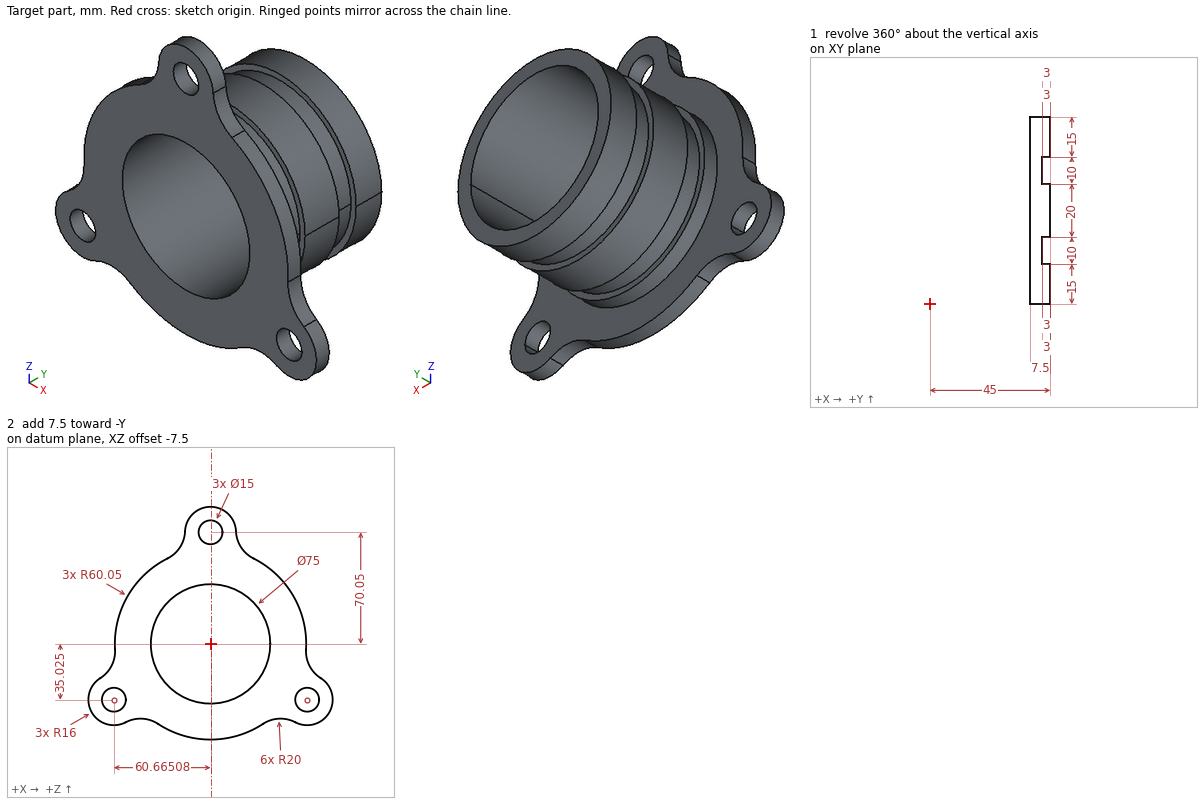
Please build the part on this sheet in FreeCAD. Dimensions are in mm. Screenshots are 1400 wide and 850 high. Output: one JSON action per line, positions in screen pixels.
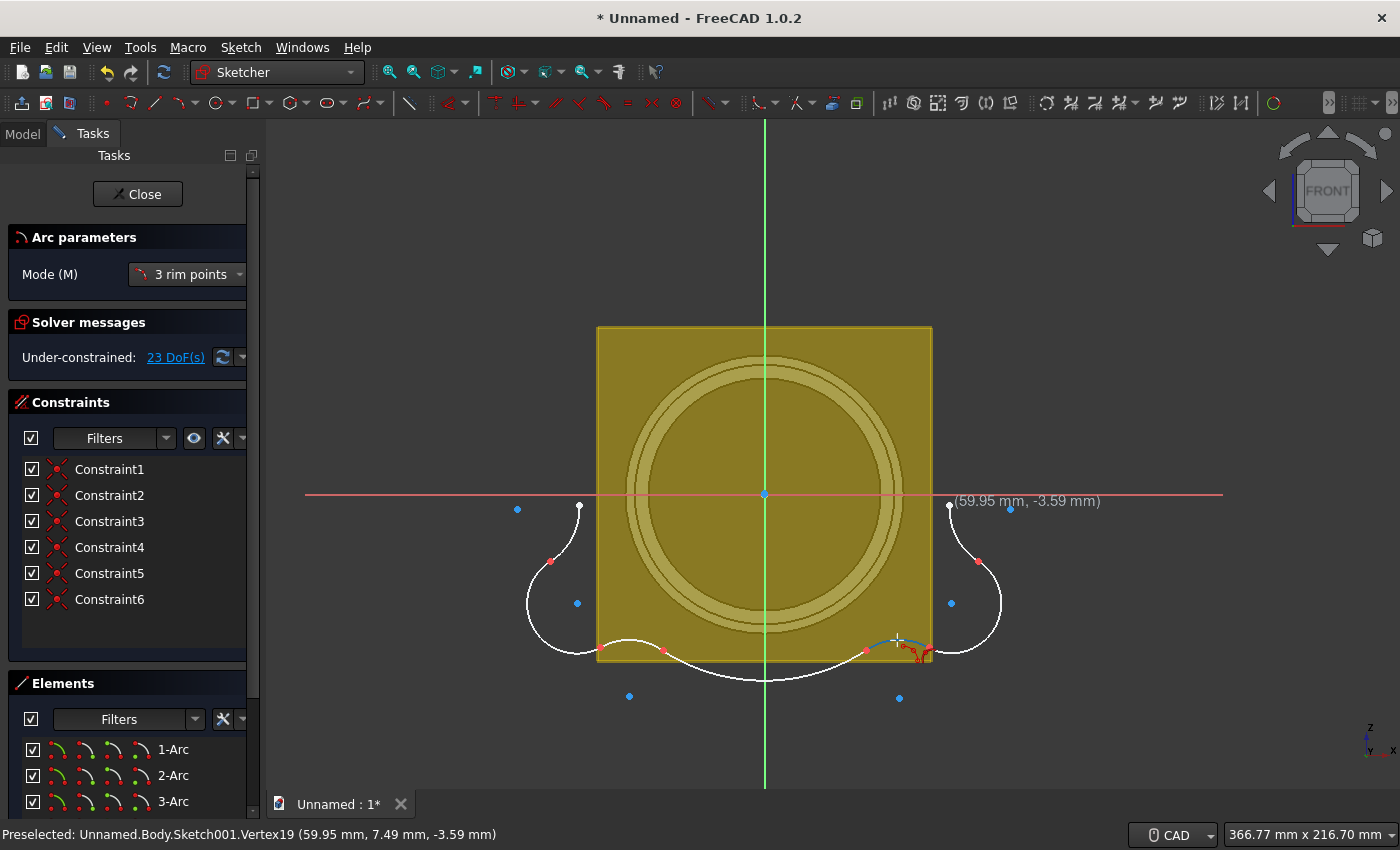
{"action": "left_click", "coordinate": [848, 329]}
{"action": "left_click", "coordinate": [925, 402]}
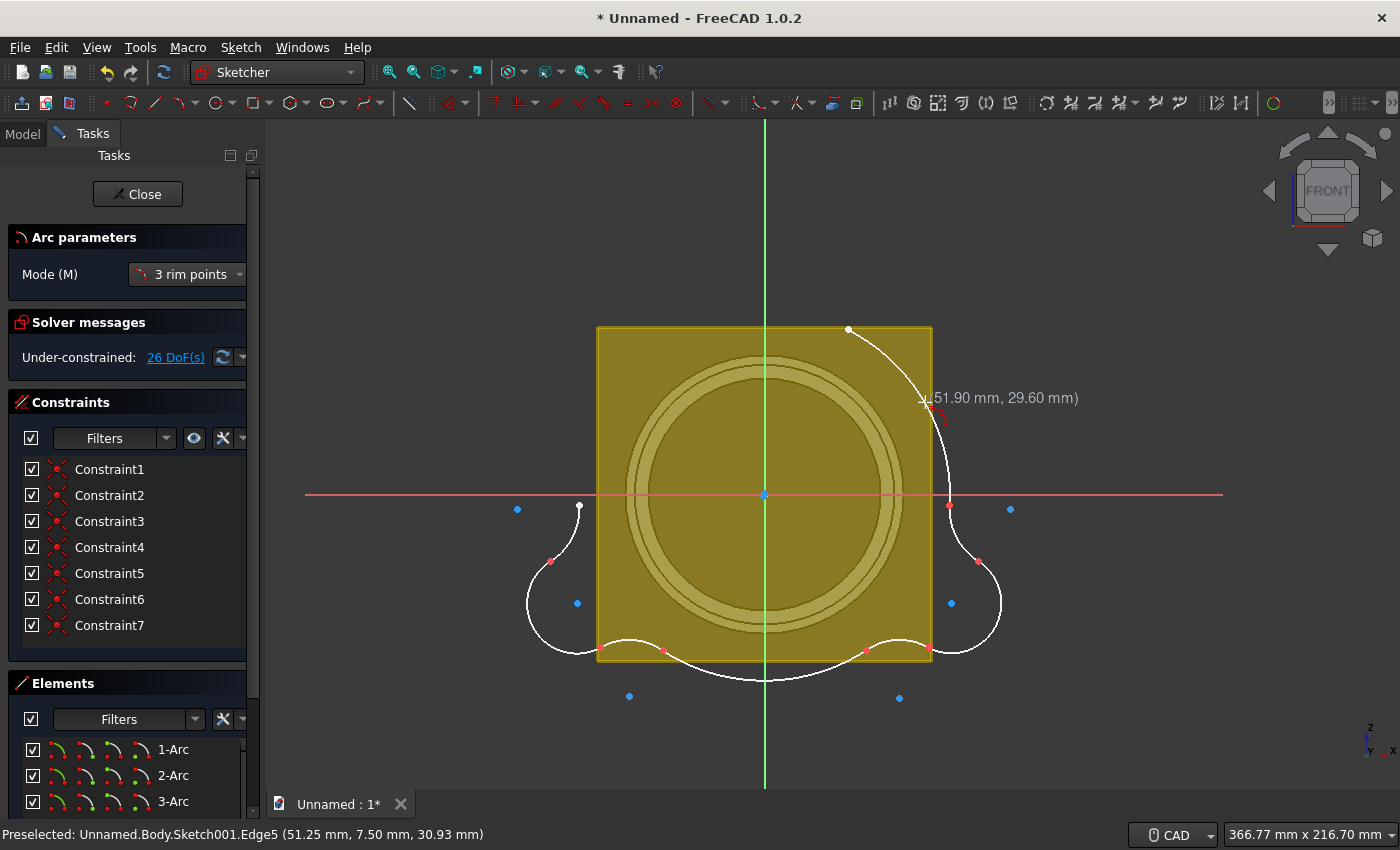
{"action": "left_click", "coordinate": [848, 330]}
{"action": "left_click", "coordinate": [814, 276]}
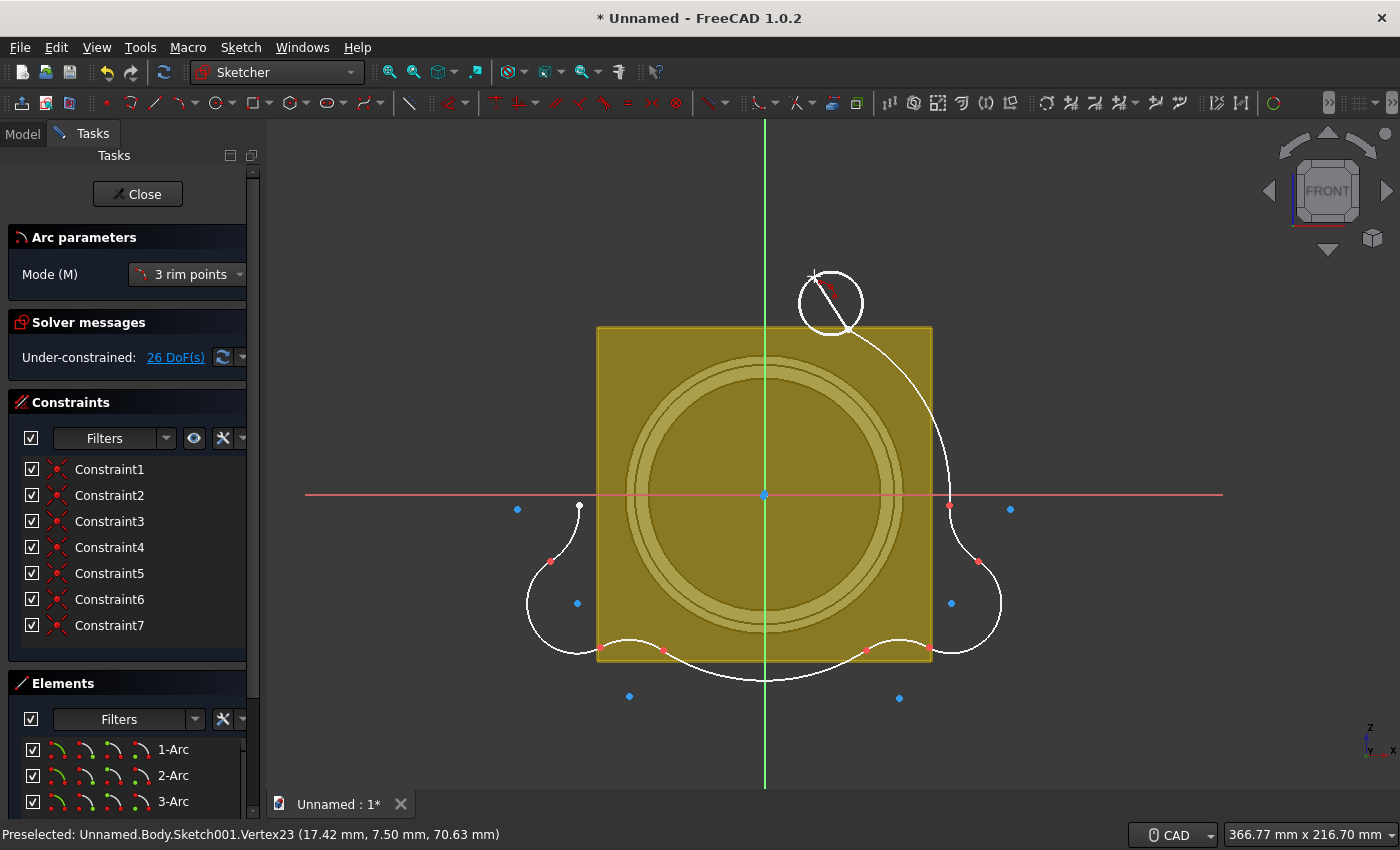
{"action": "scroll", "coordinate": [824, 307], "scroll_direction": "up", "scroll_amount": 4}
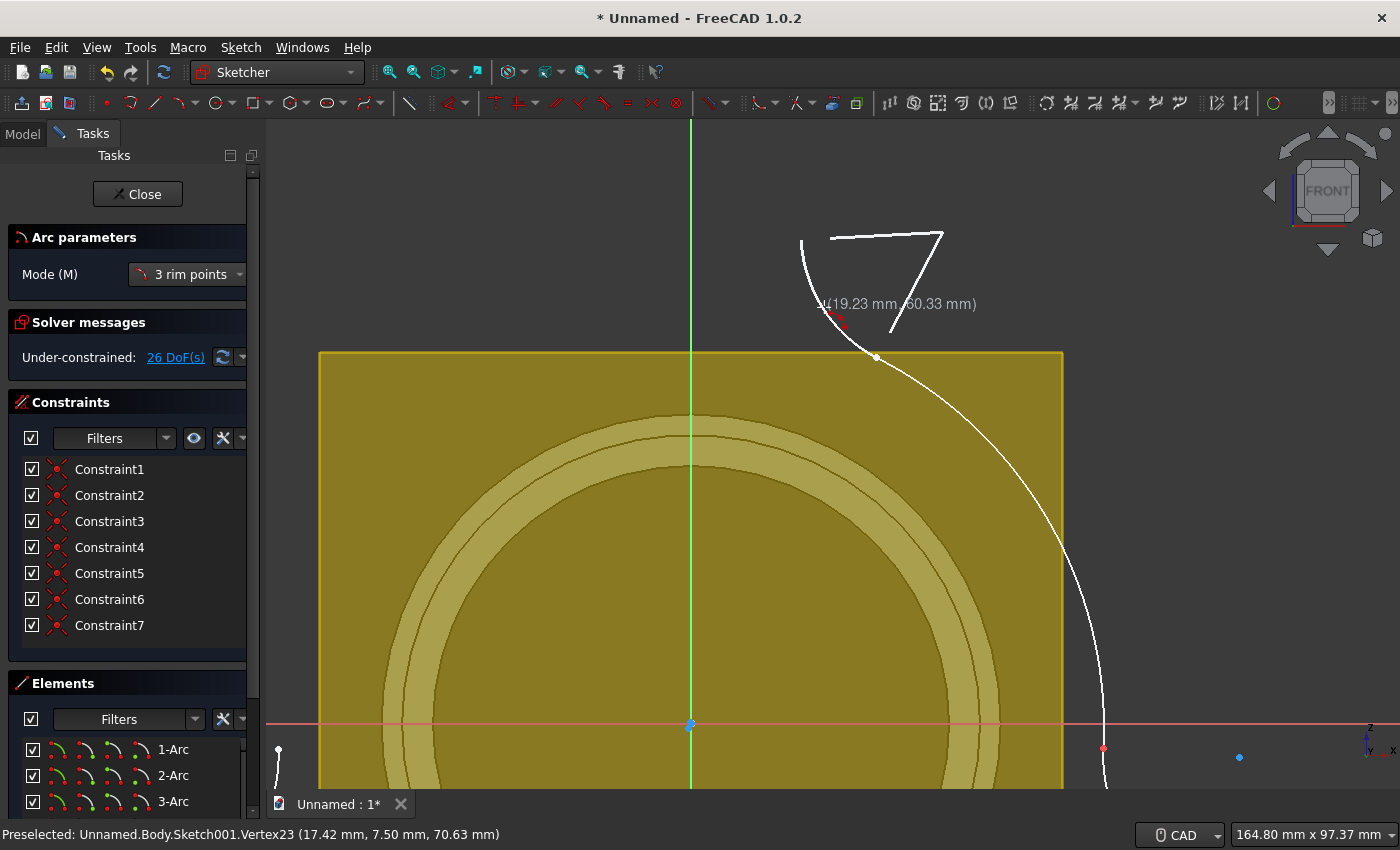
{"action": "left_click", "coordinate": [823, 306]}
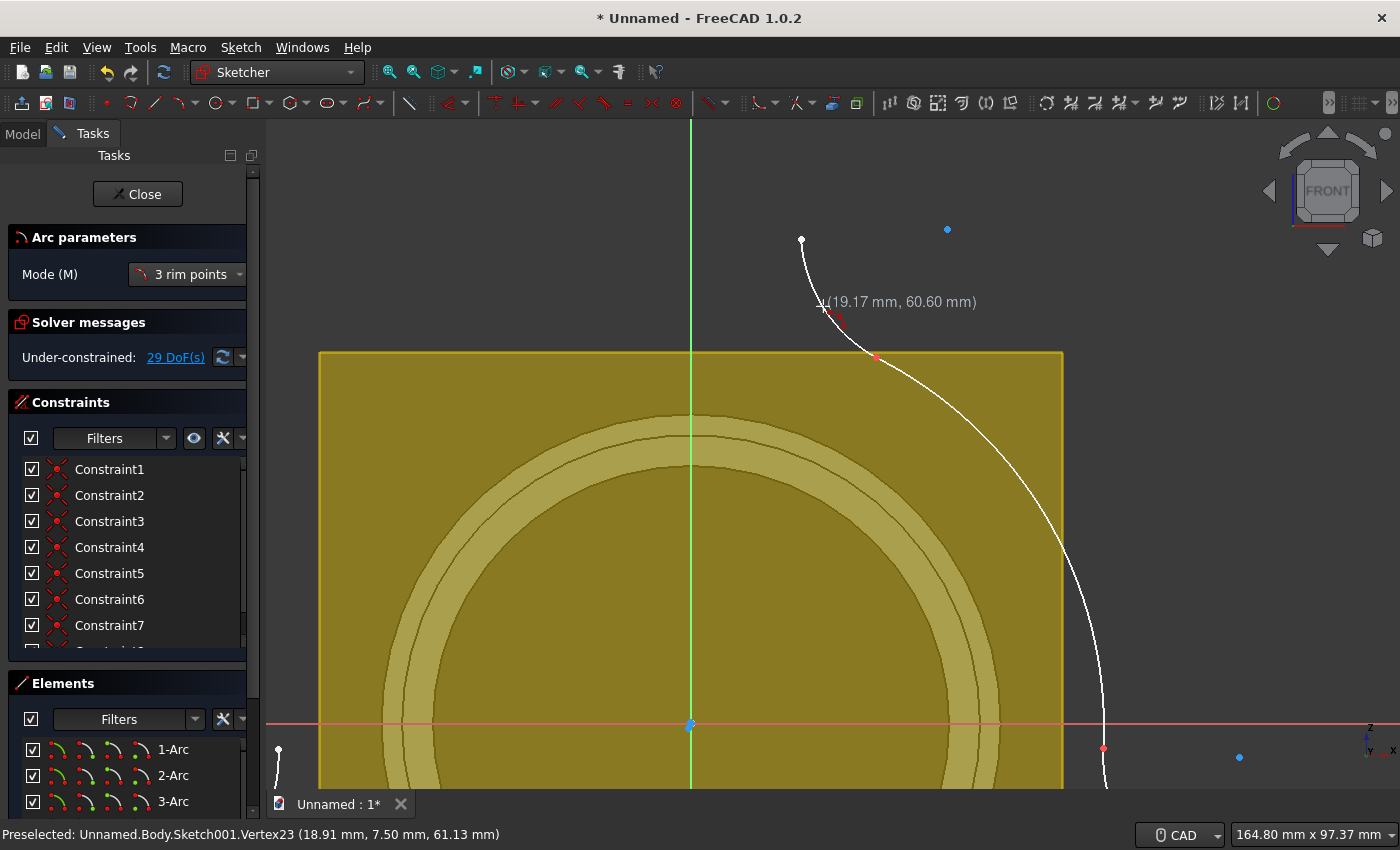
{"action": "left_click", "coordinate": [801, 240]}
{"action": "left_click", "coordinate": [581, 238]}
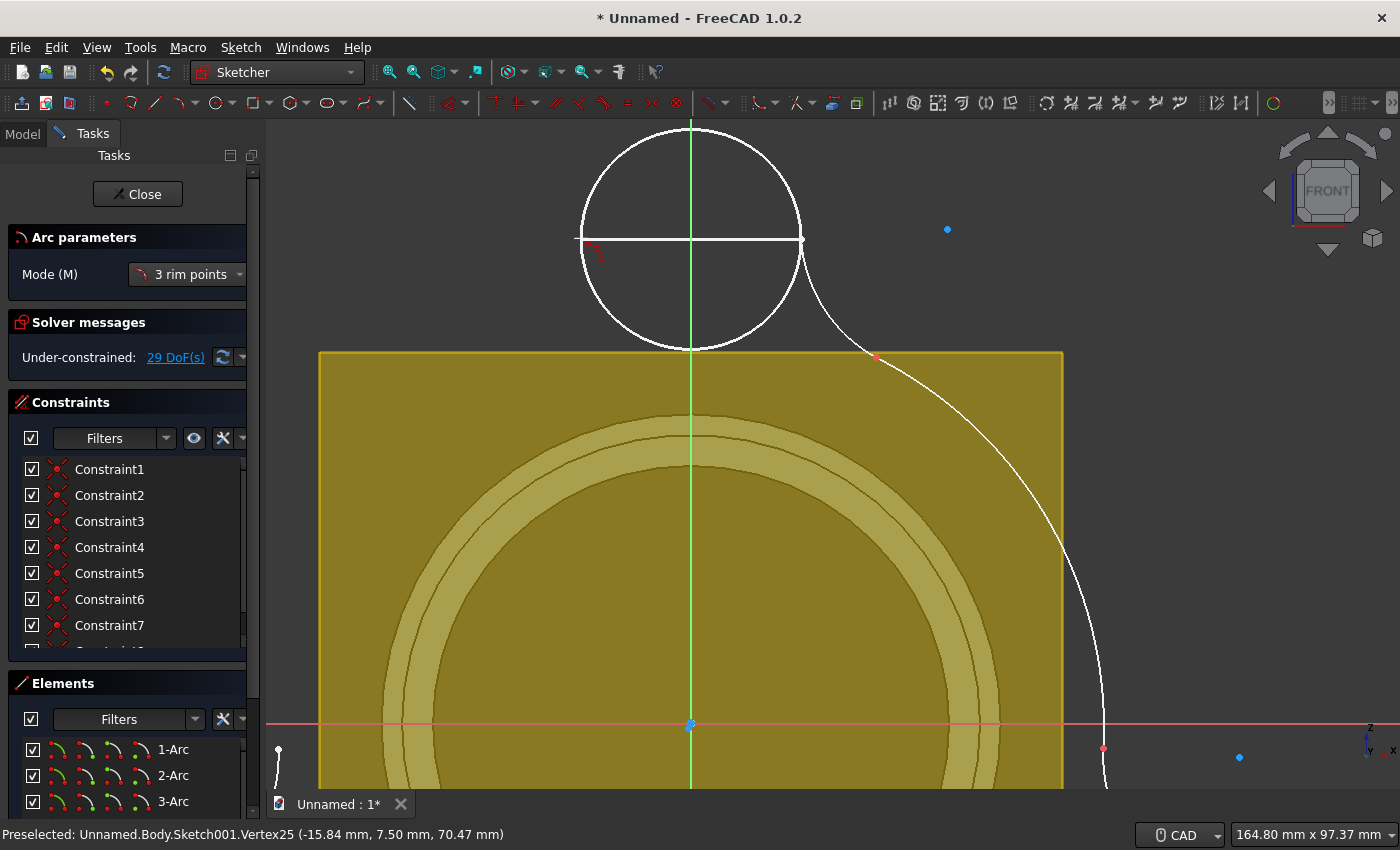
{"action": "scroll", "coordinate": [824, 307], "scroll_direction": "down", "scroll_amount": 4}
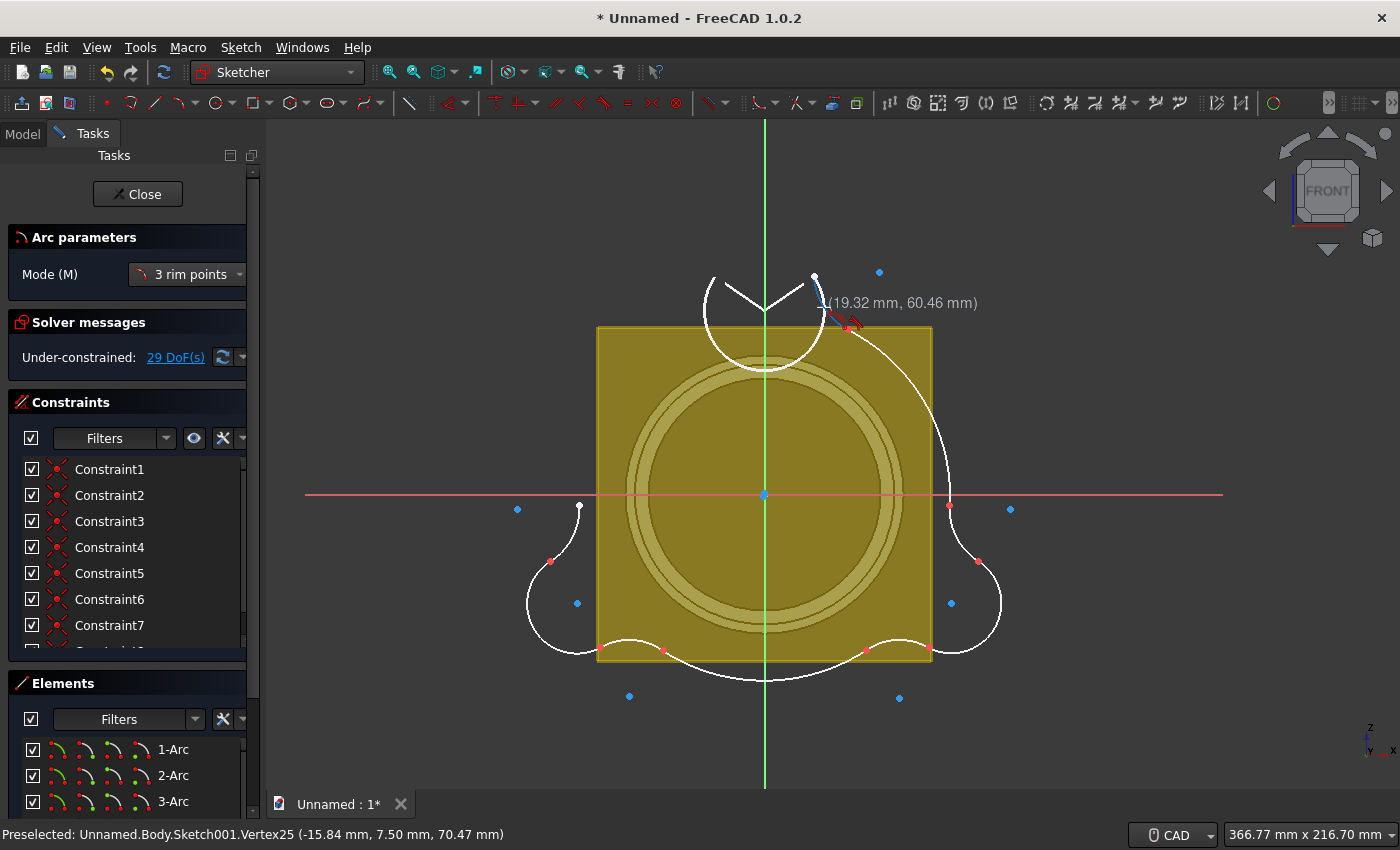
{"action": "left_click", "coordinate": [779, 231]}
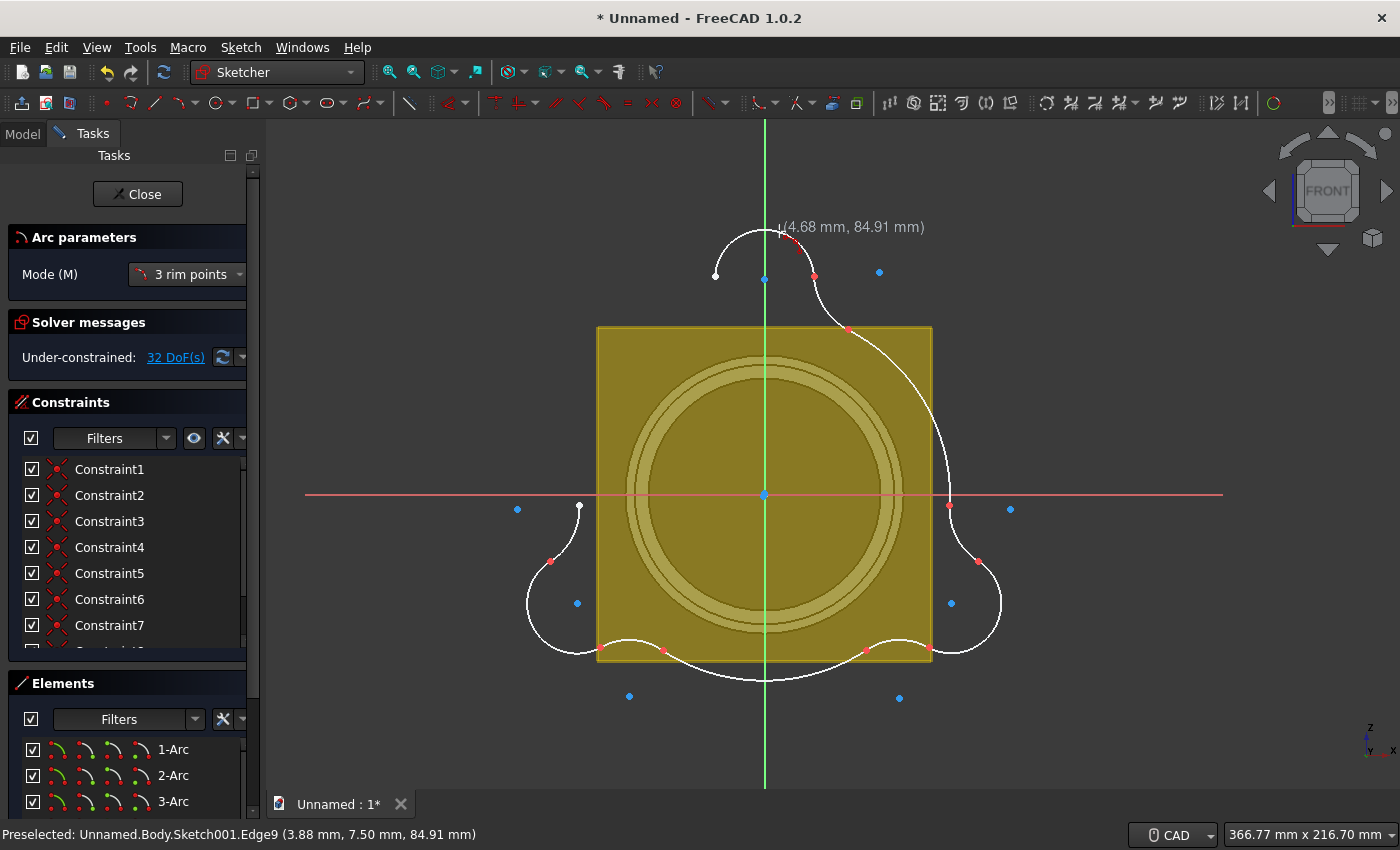
{"action": "left_click", "coordinate": [715, 277]}
{"action": "left_click", "coordinate": [681, 329]}